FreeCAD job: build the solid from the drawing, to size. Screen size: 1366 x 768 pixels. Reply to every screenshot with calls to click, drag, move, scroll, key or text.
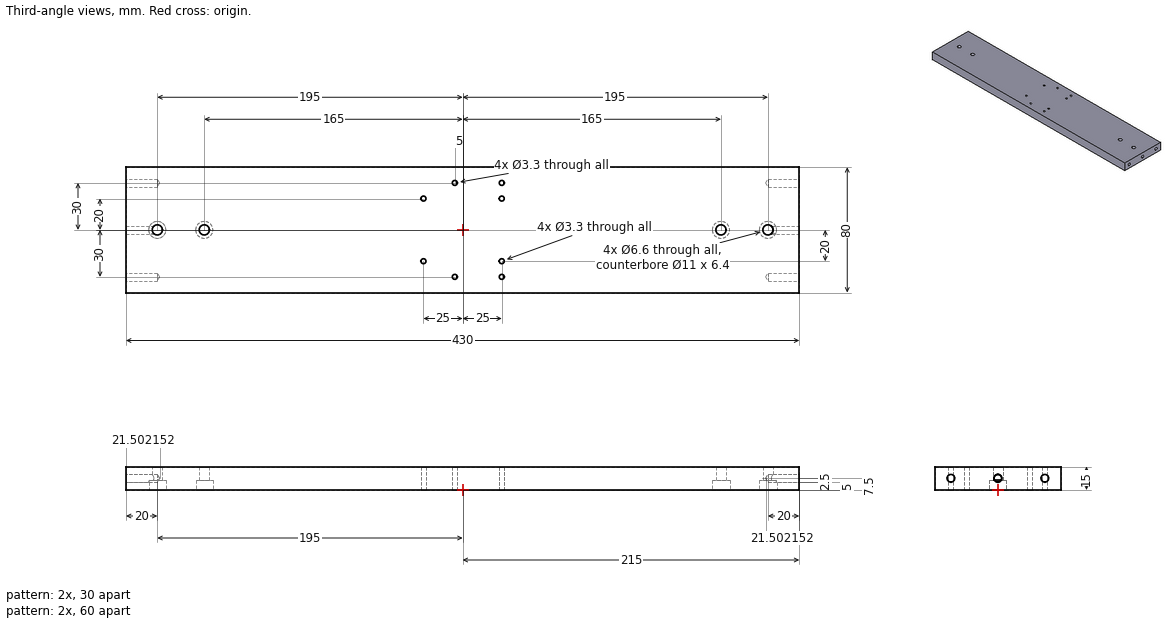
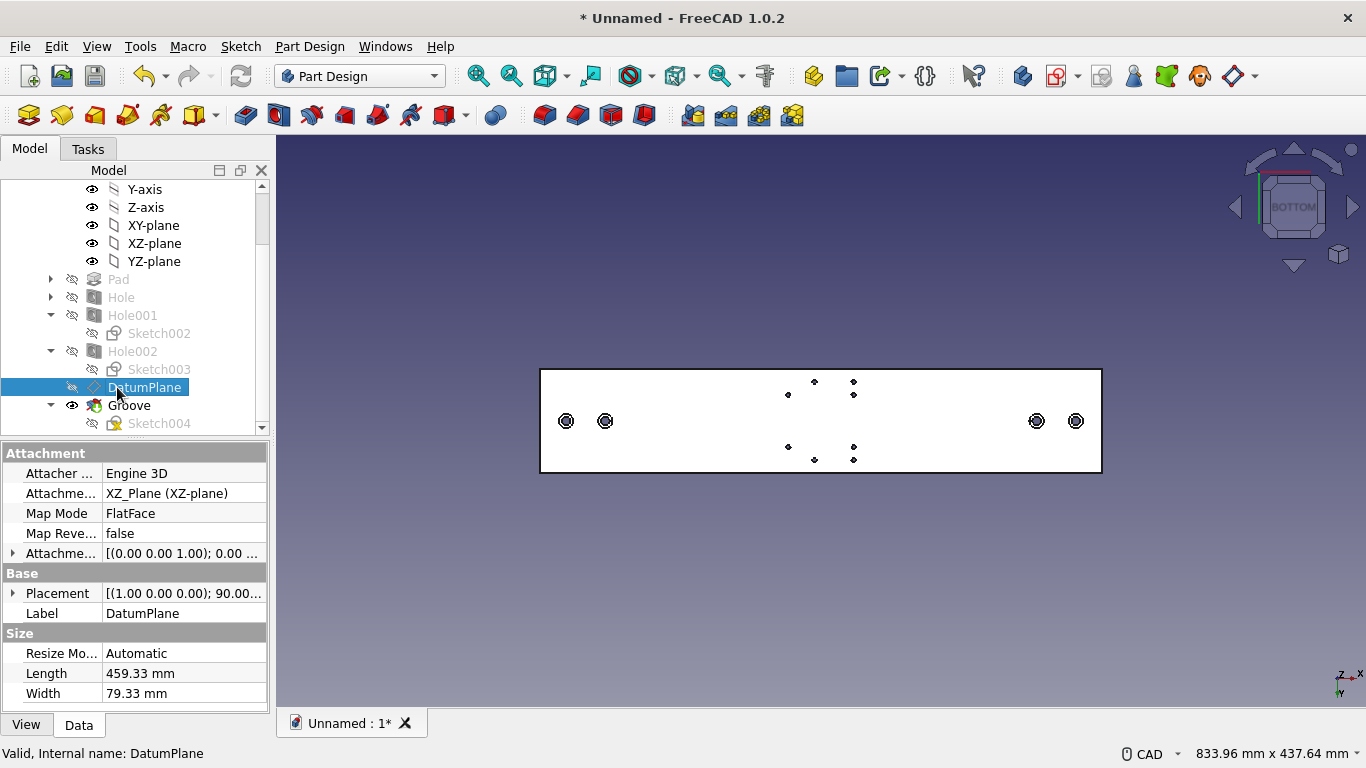
click(117, 405)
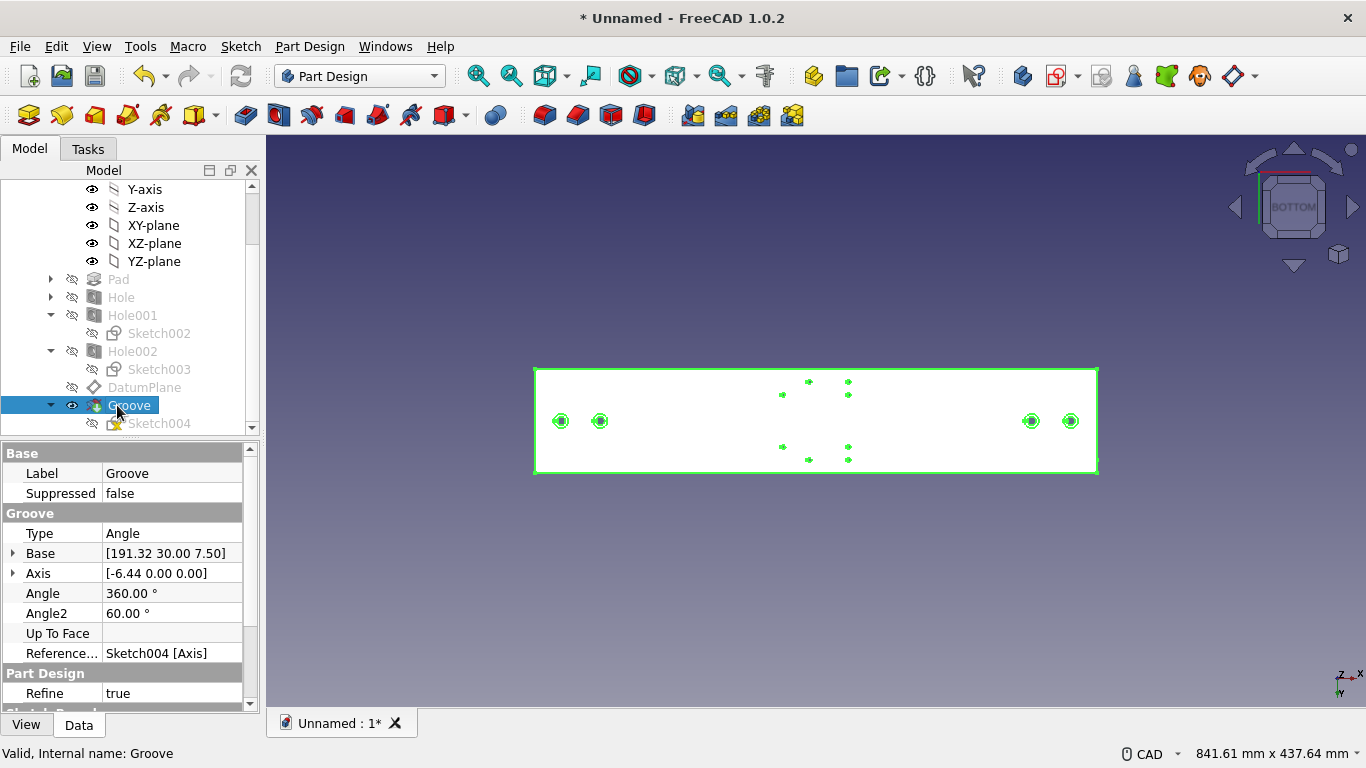
click(726, 116)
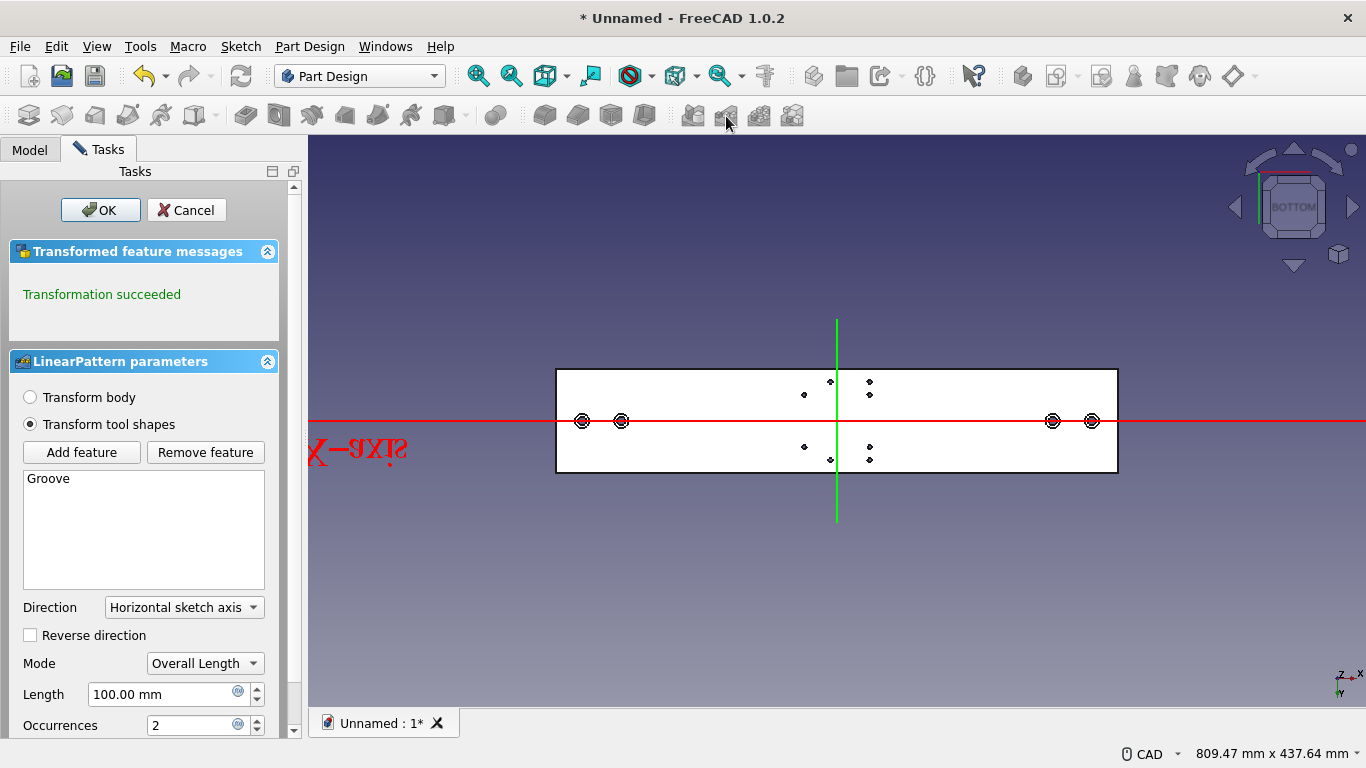
click(185, 608)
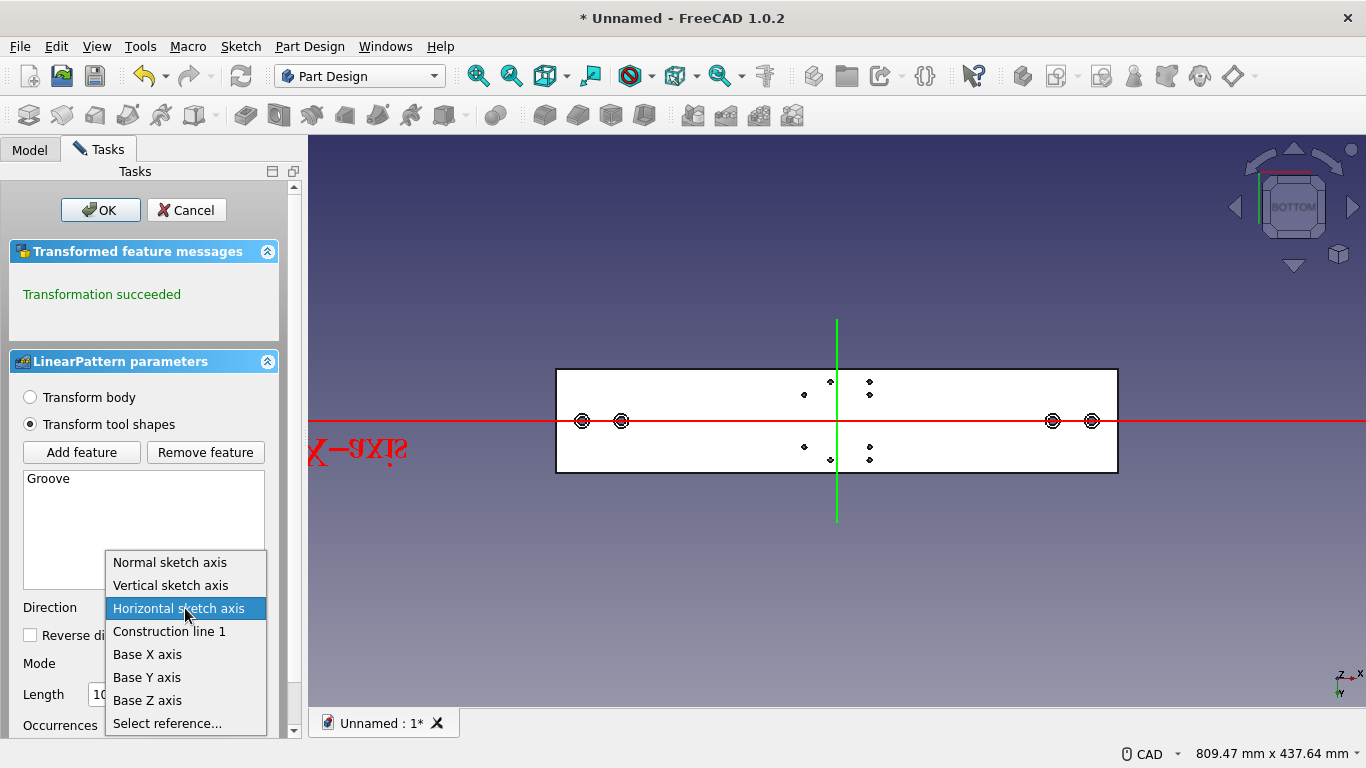
click(184, 678)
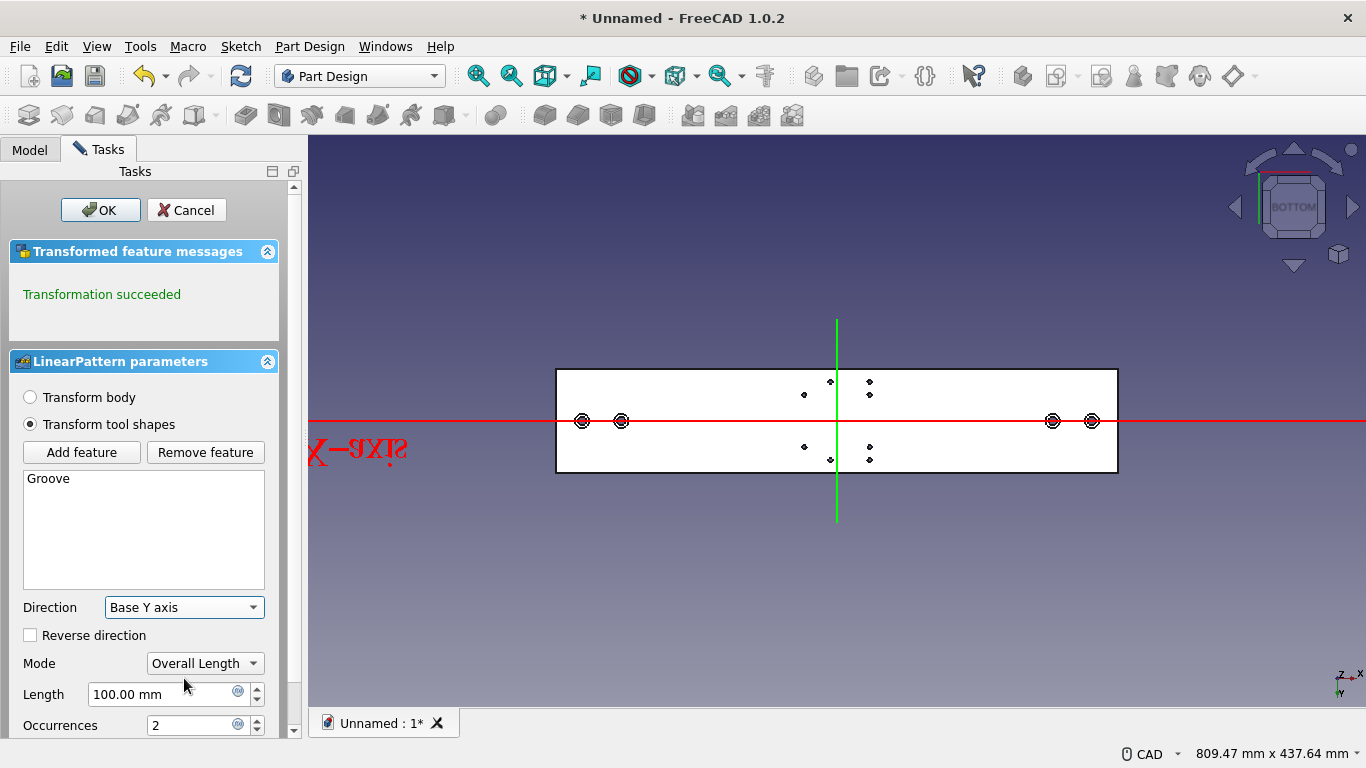
click(206, 664)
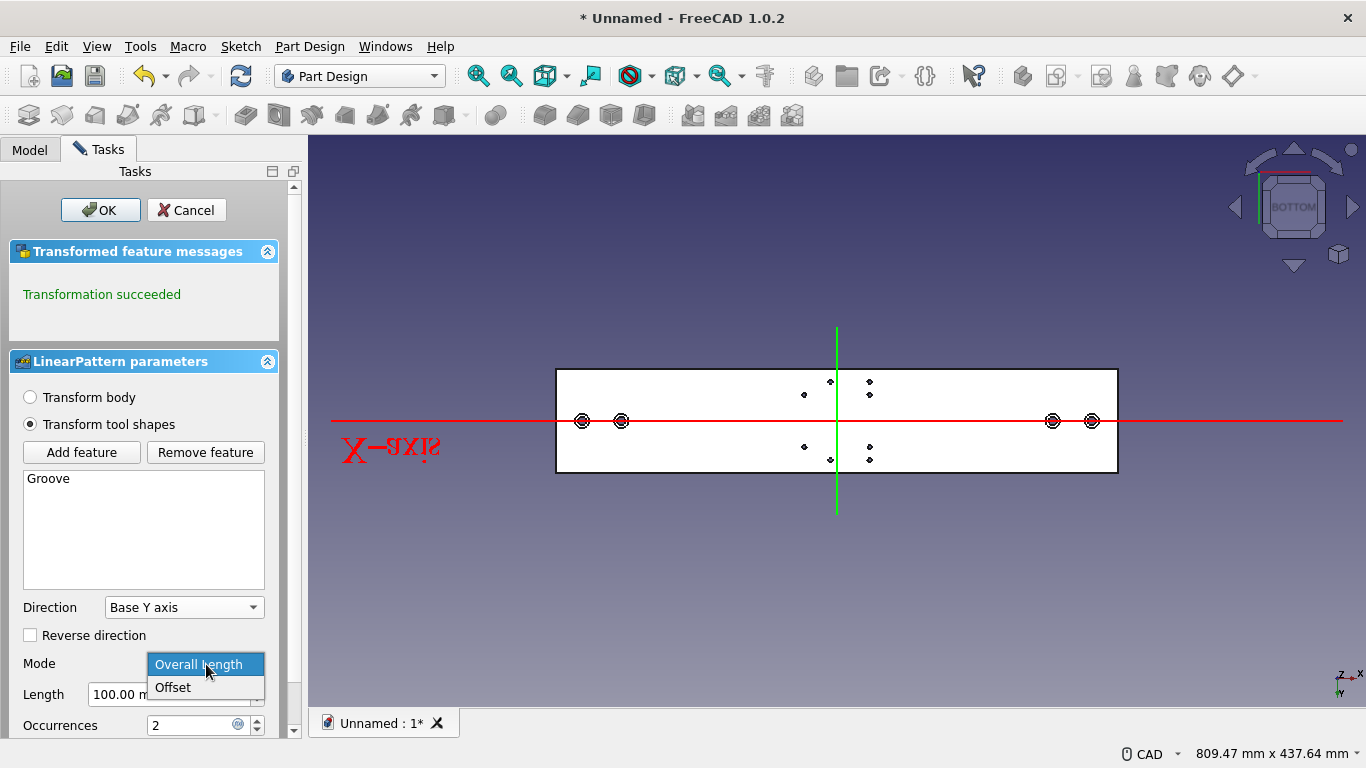
click(204, 688)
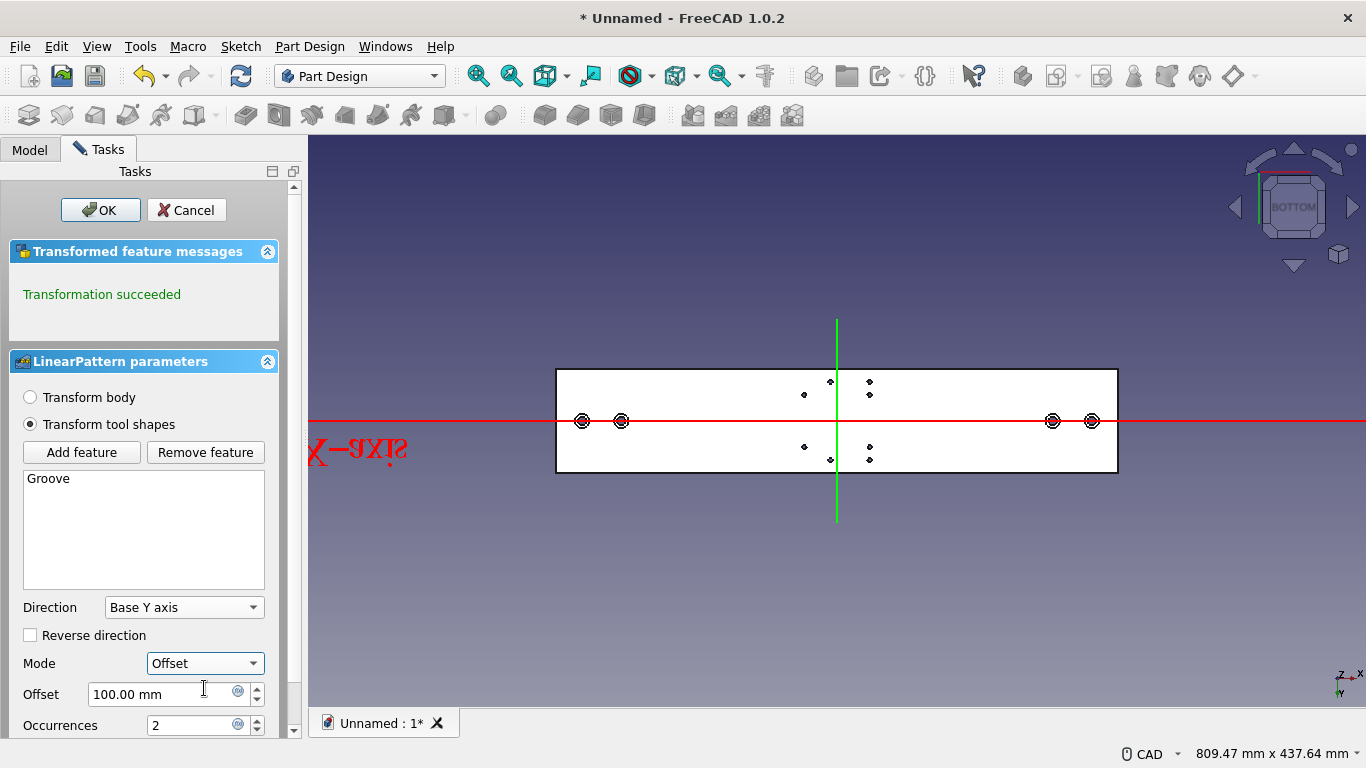
triple_click(170, 694)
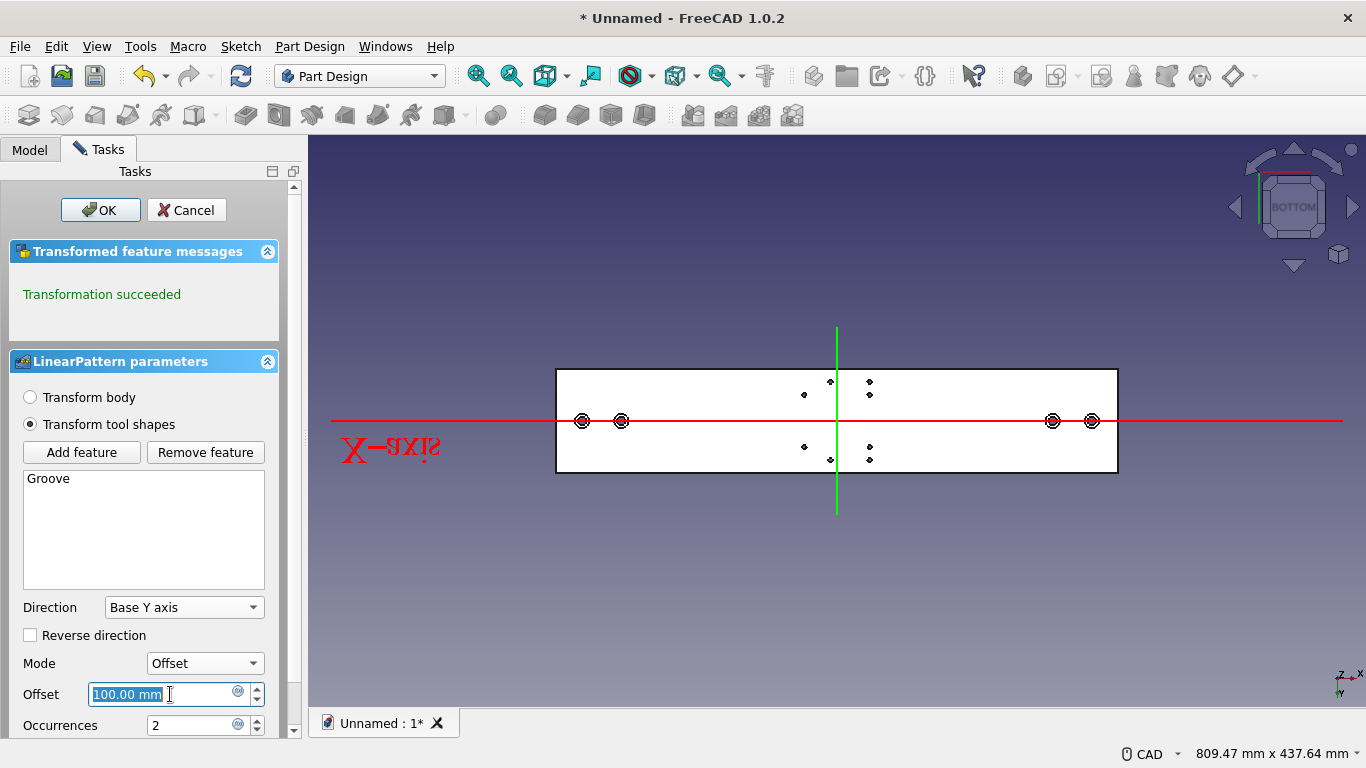
text(30)
key(Tab)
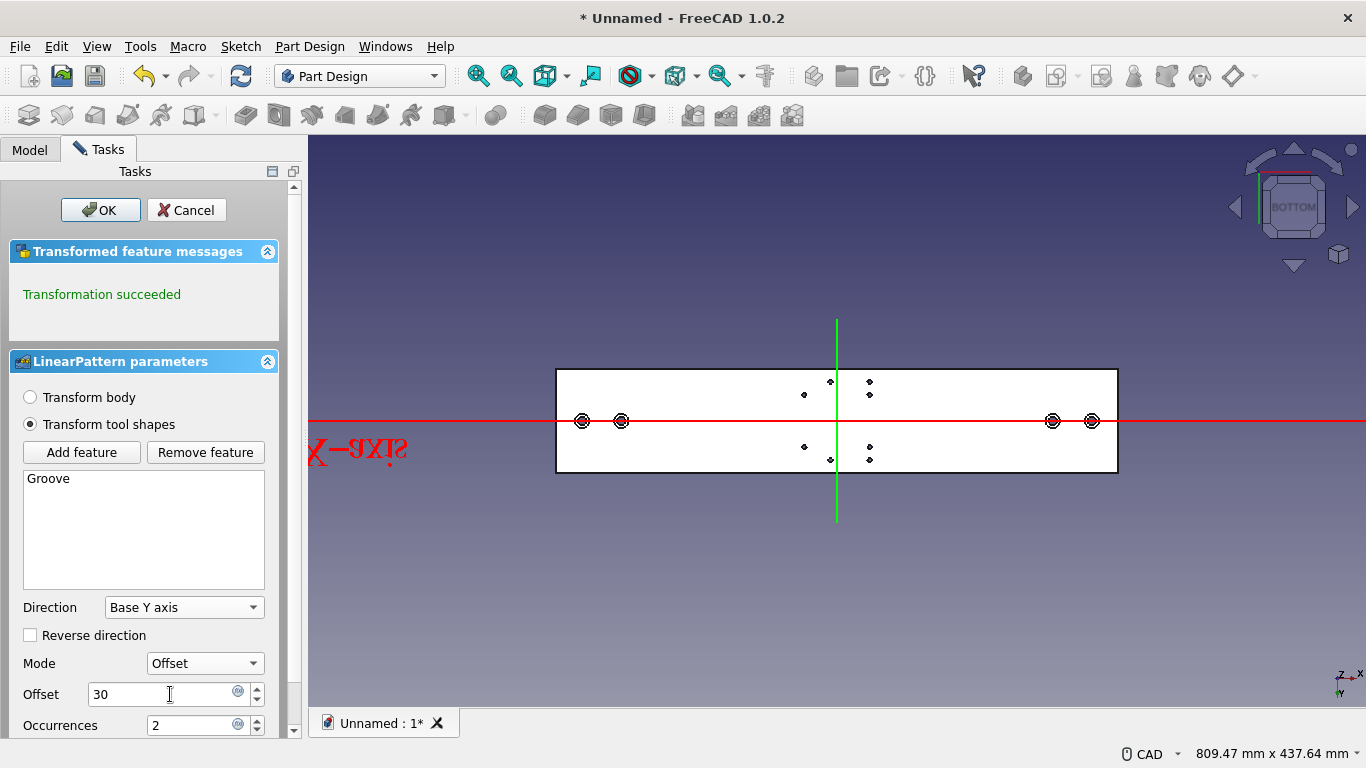
triple_click(199, 726)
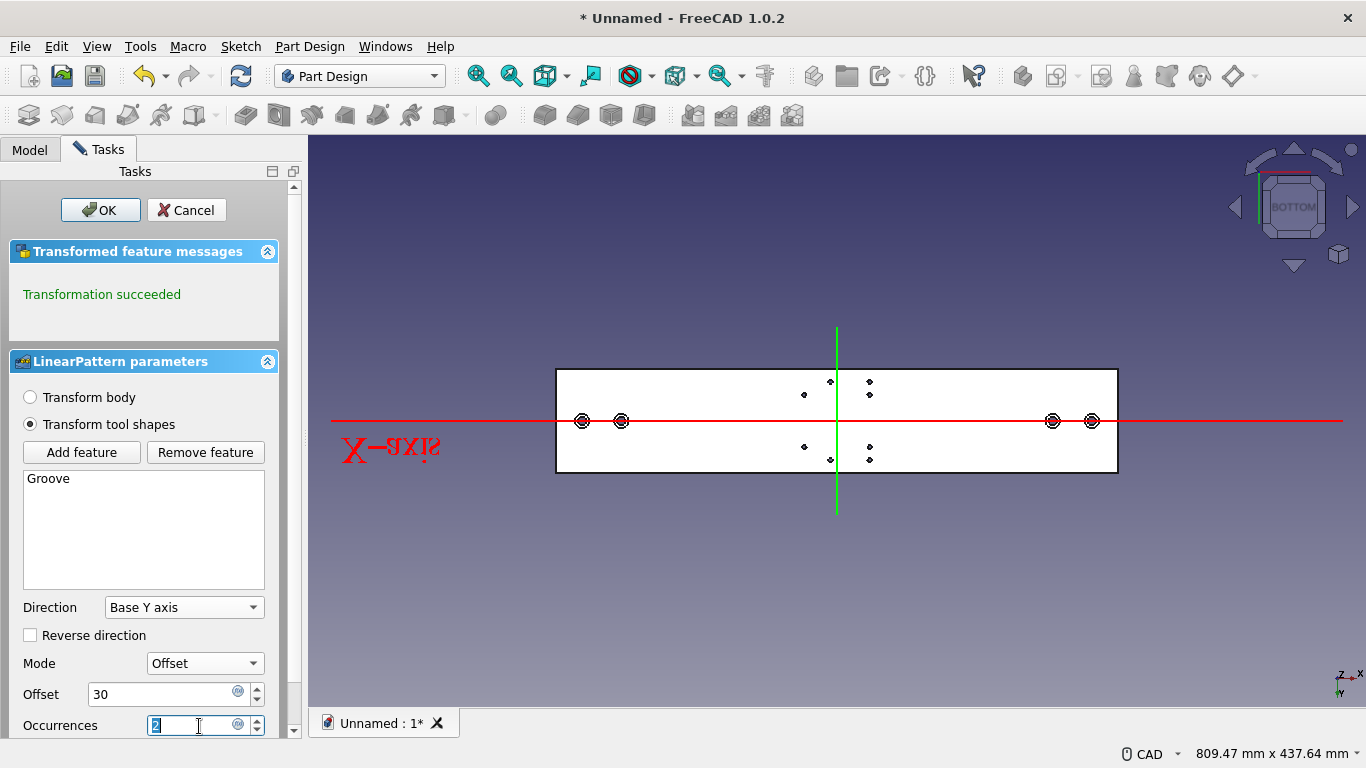
text(2)
key(Tab)